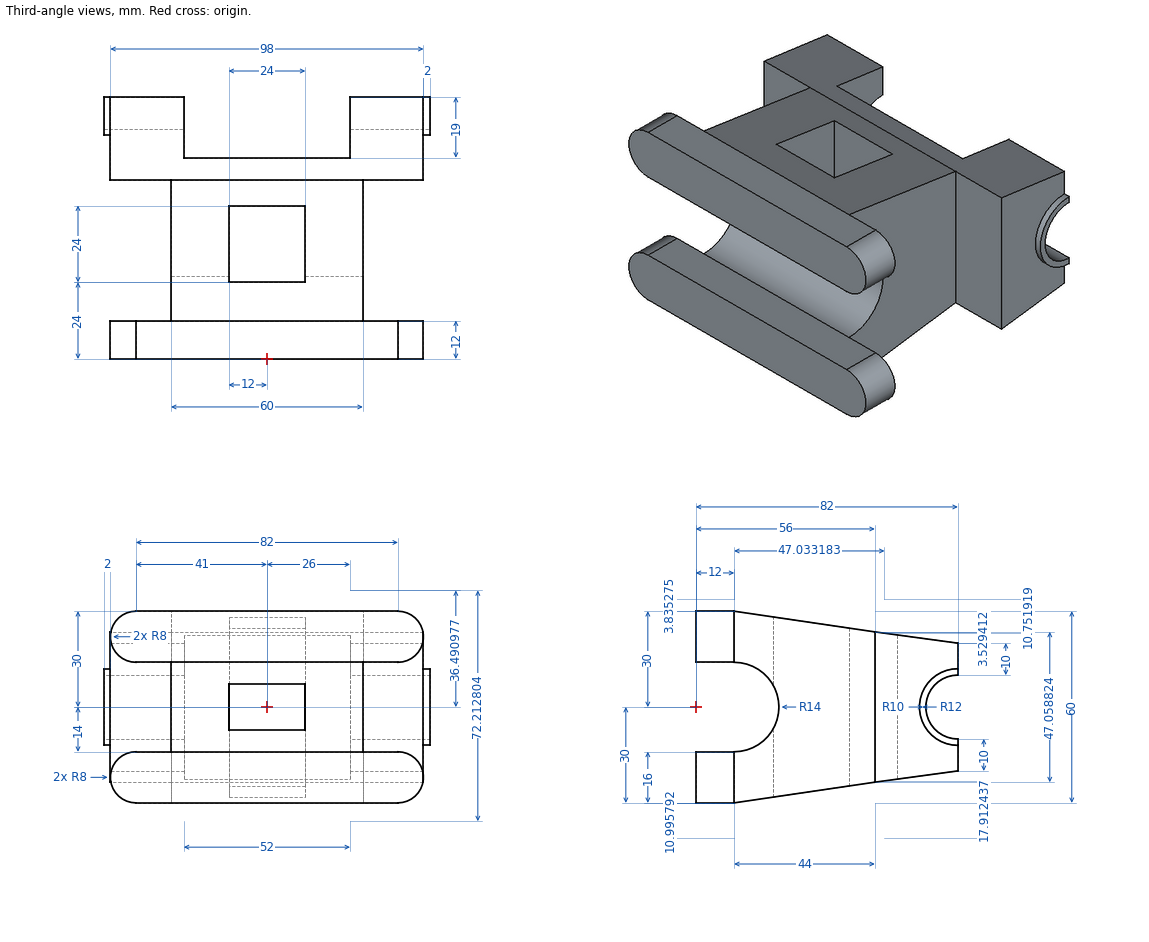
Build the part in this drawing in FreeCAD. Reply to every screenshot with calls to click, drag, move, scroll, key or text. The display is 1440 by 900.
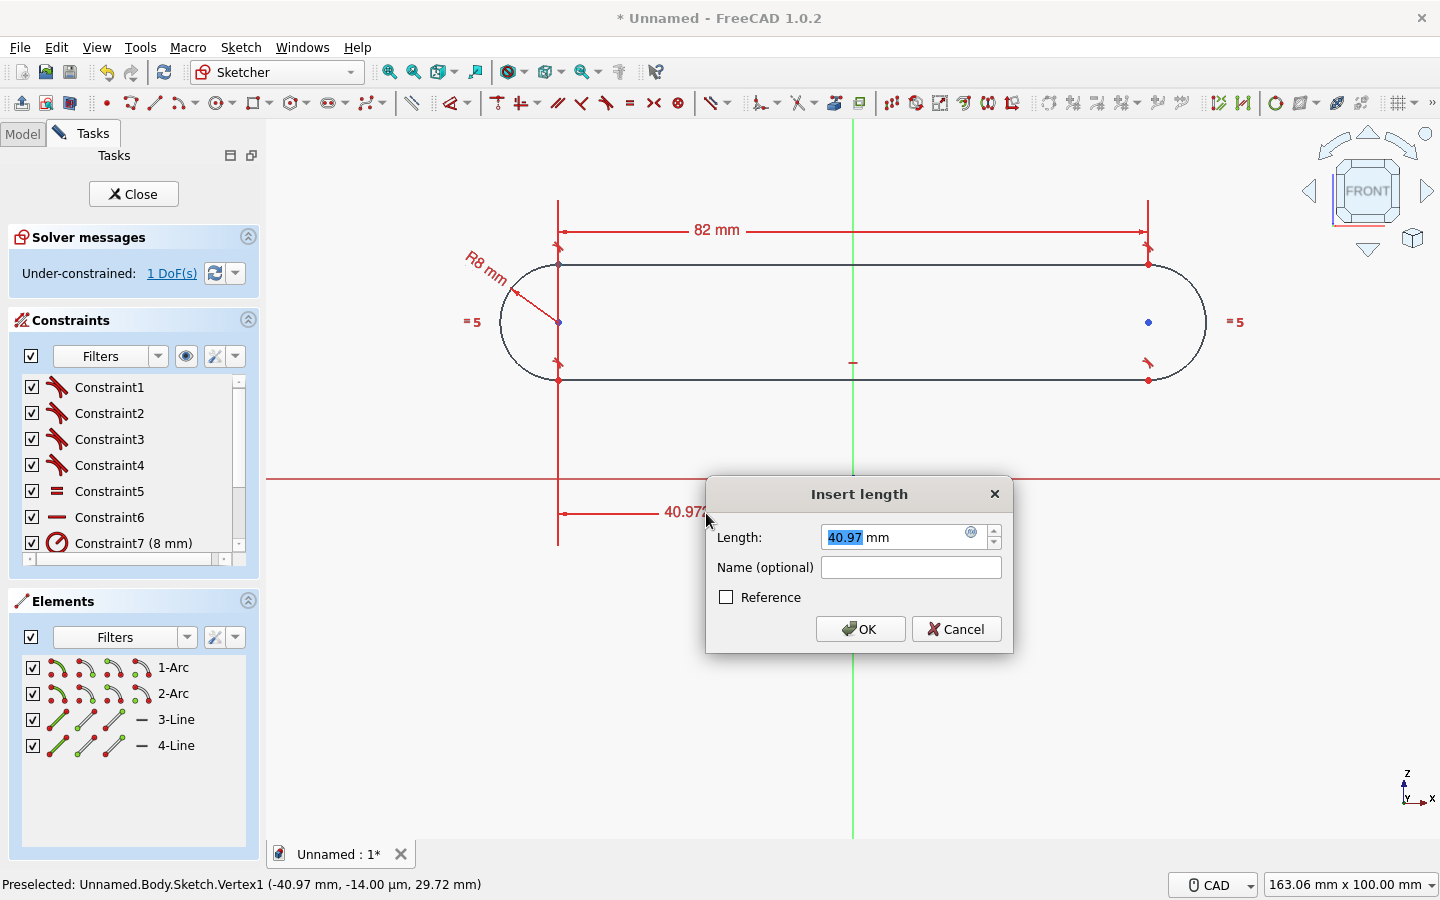
text(41)
key(Return)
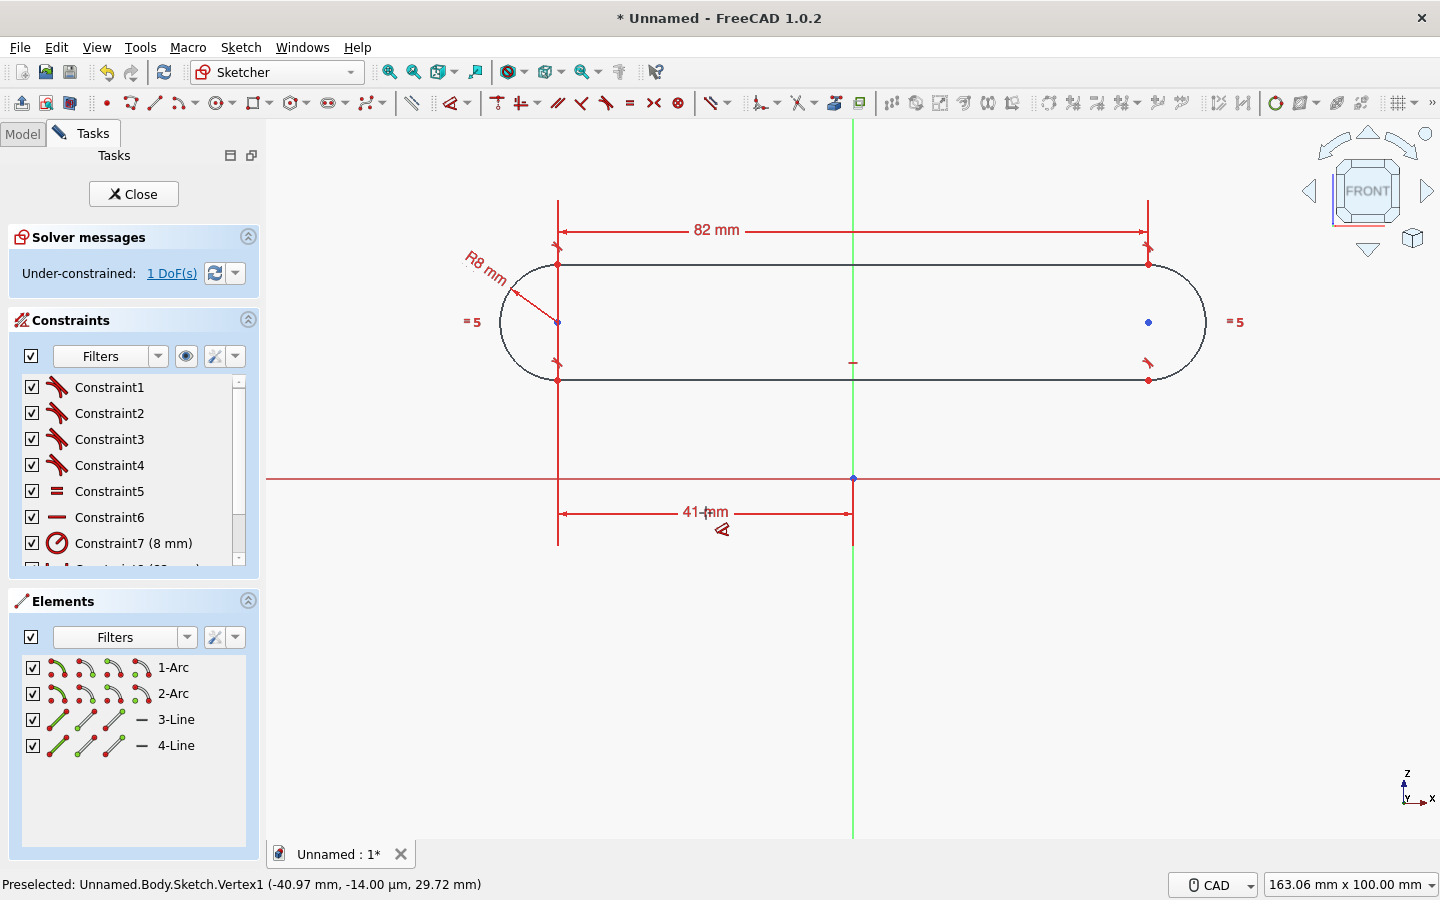
click(558, 265)
click(524, 323)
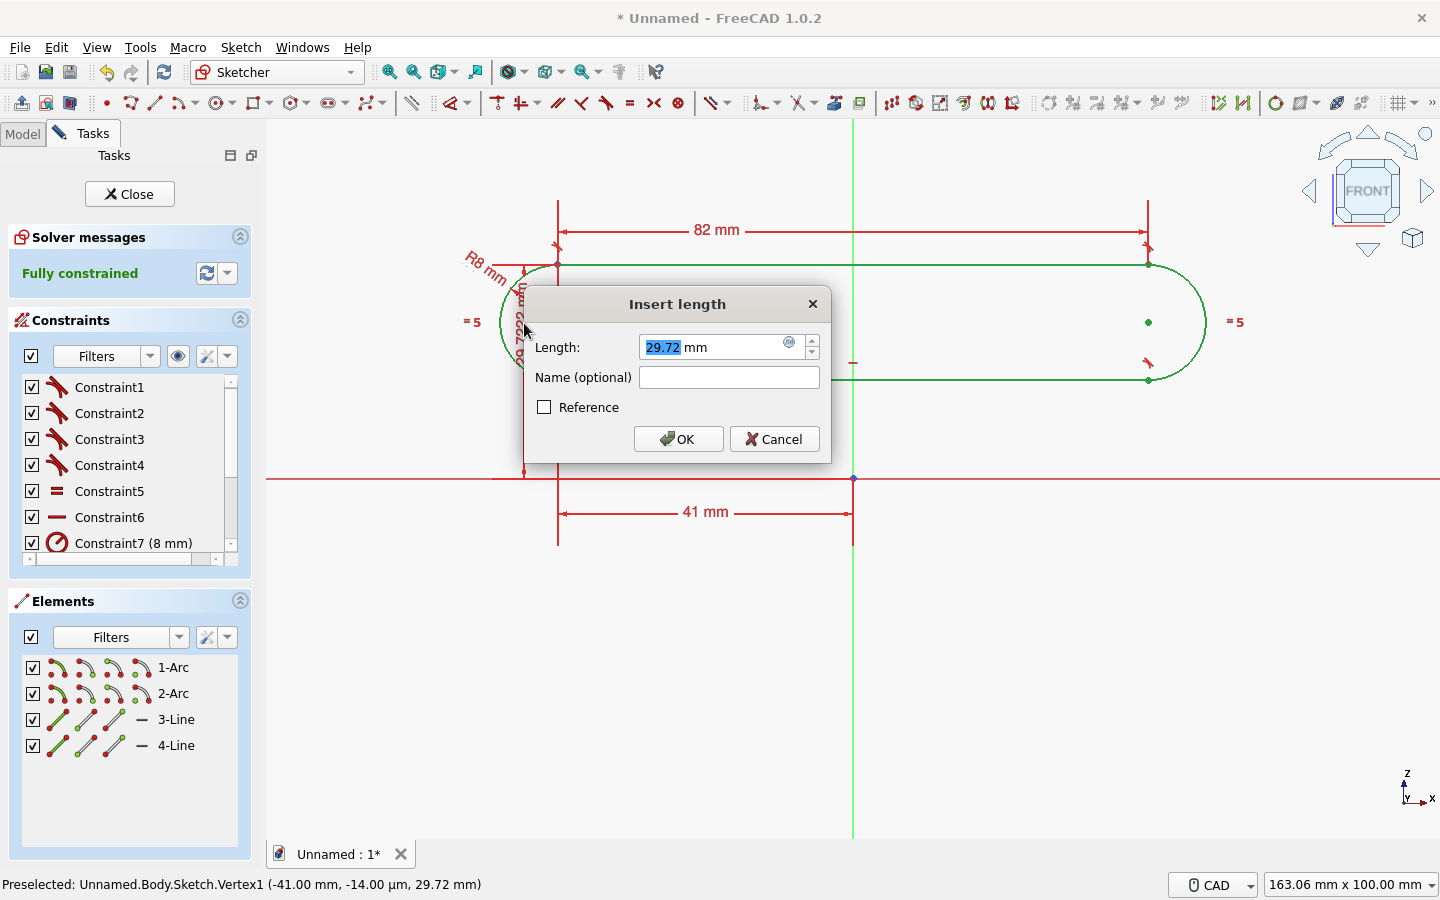
text(30)
key(Return)
key(Escape)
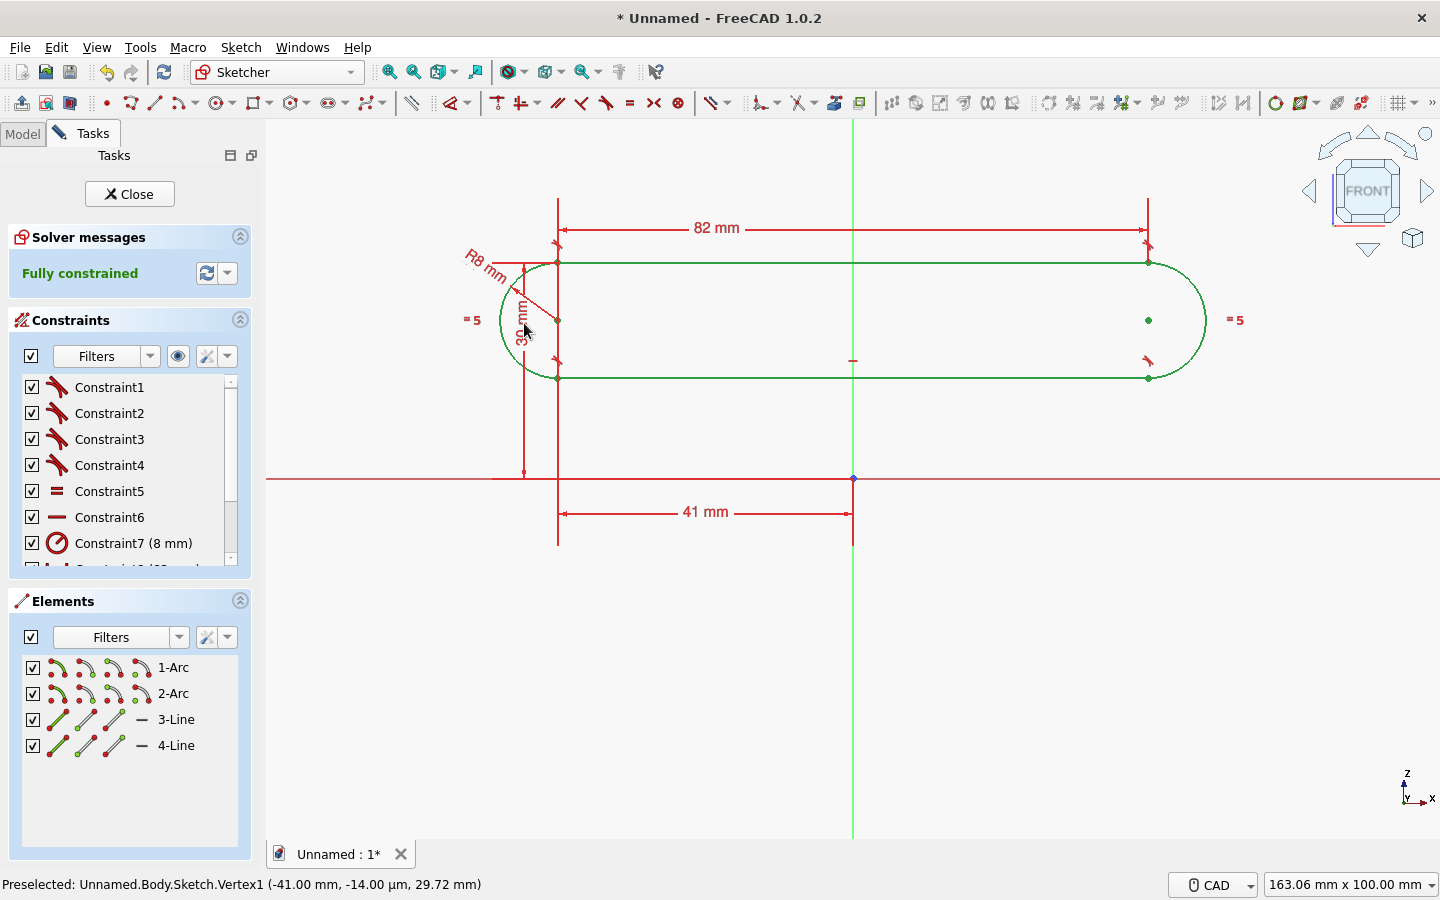
click(130, 194)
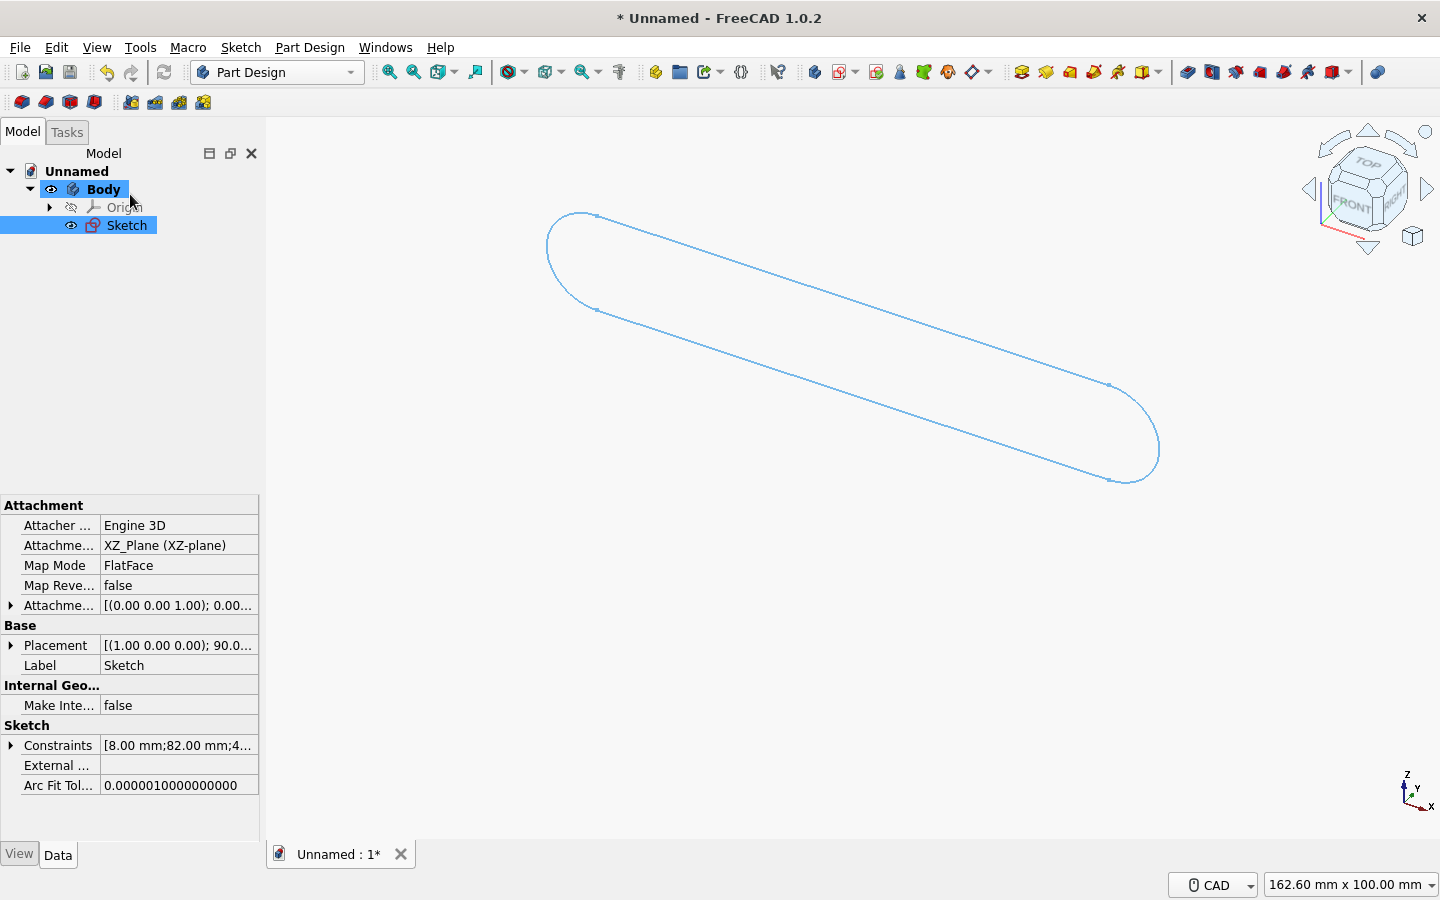
click(1022, 72)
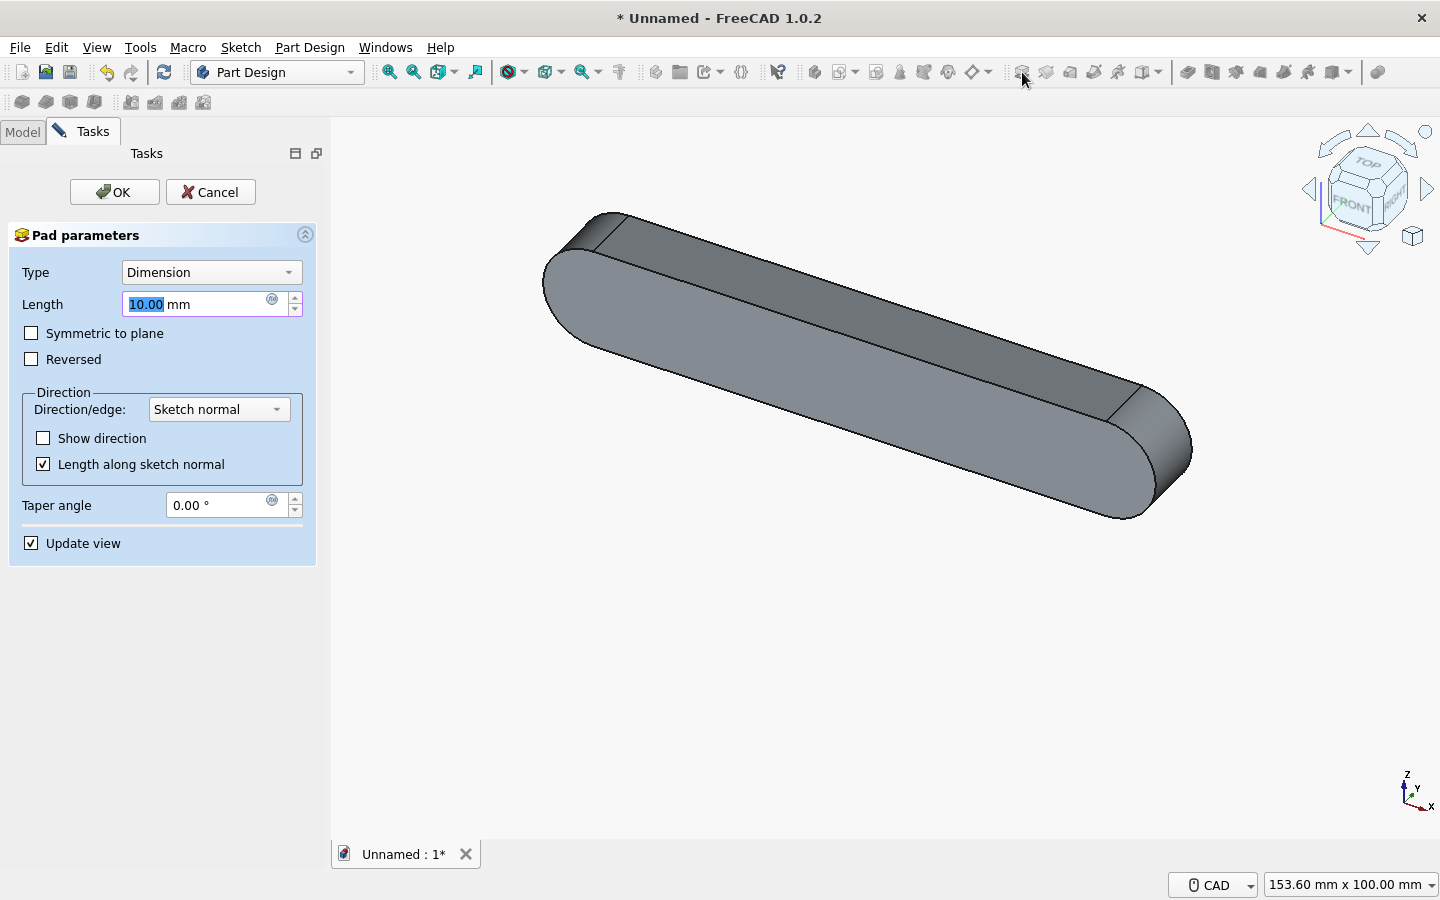
text(12)
key(Tab)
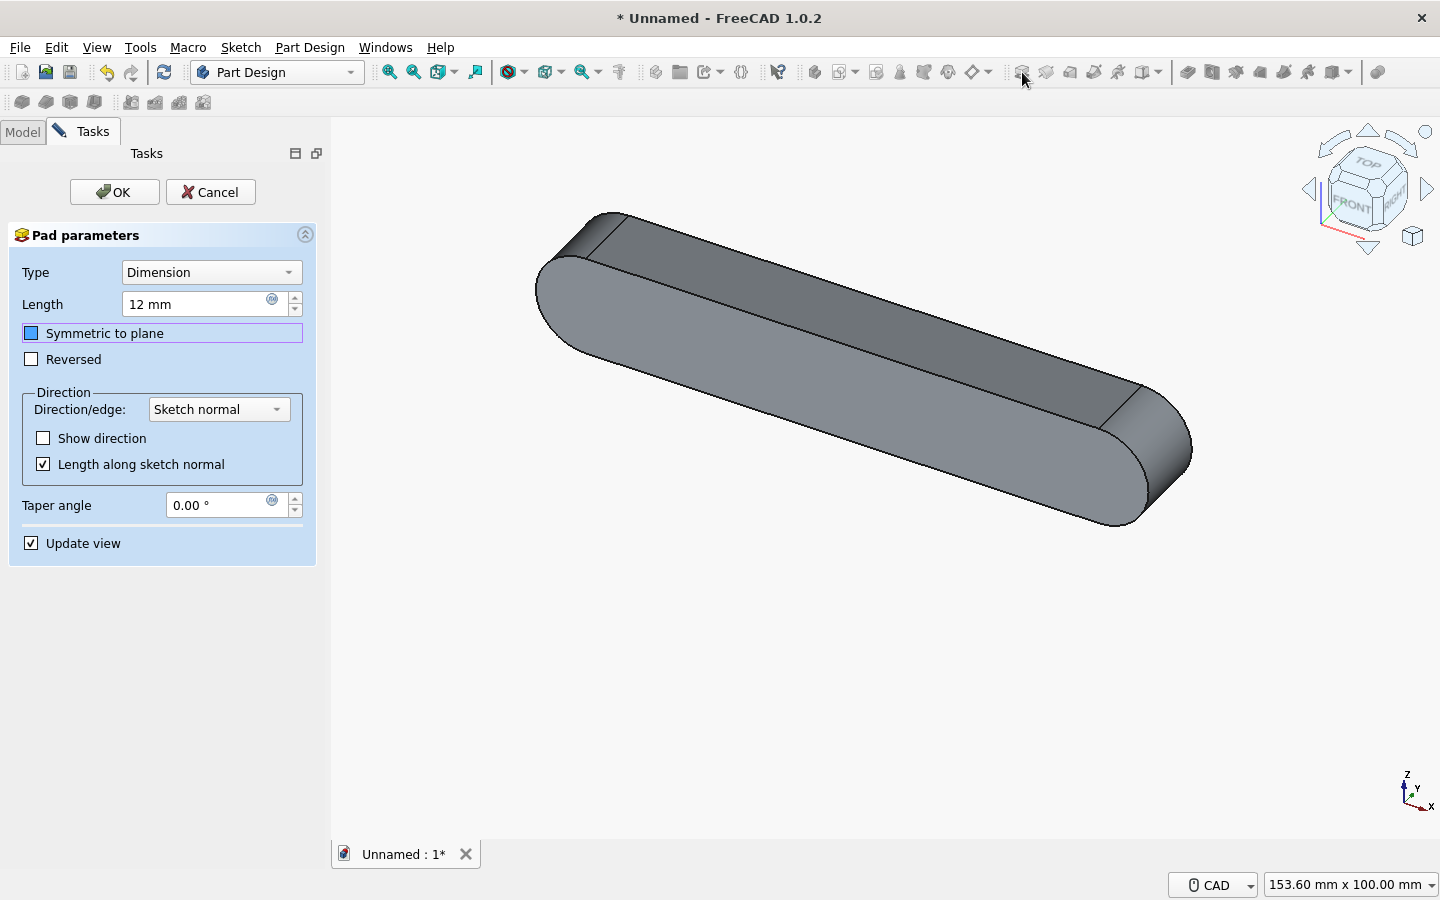
click(30, 359)